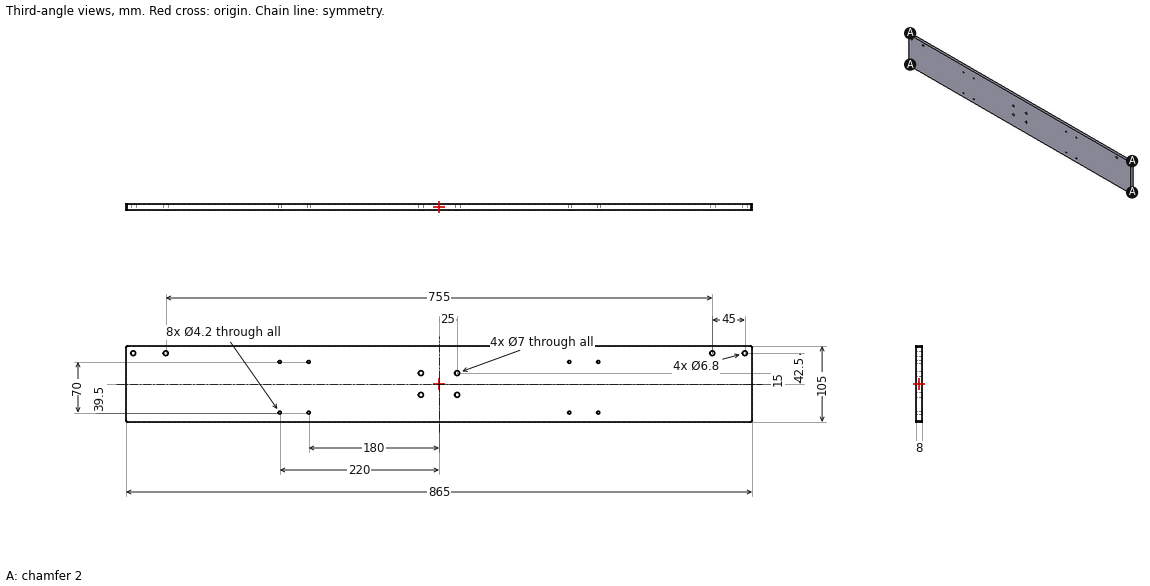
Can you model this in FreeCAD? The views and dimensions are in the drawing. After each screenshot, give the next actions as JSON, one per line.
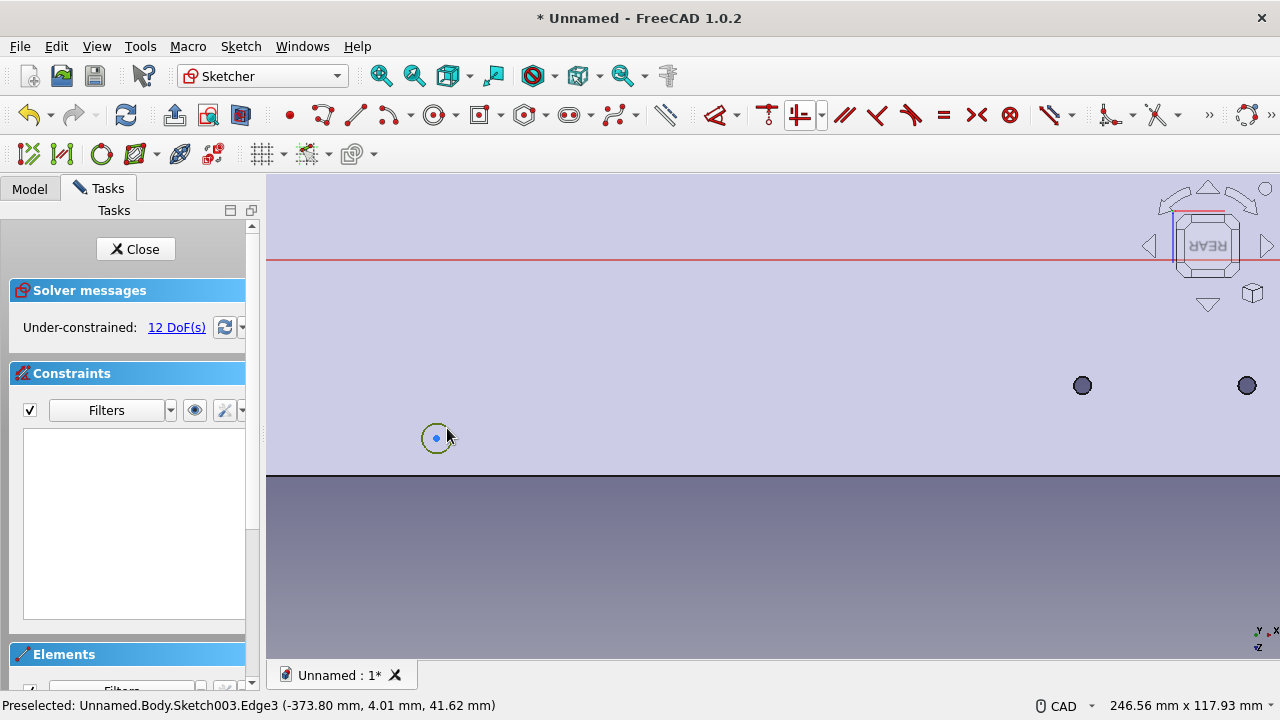
{"action": "scroll", "coordinate": [450, 429], "scroll_direction": "down", "scroll_amount": 9}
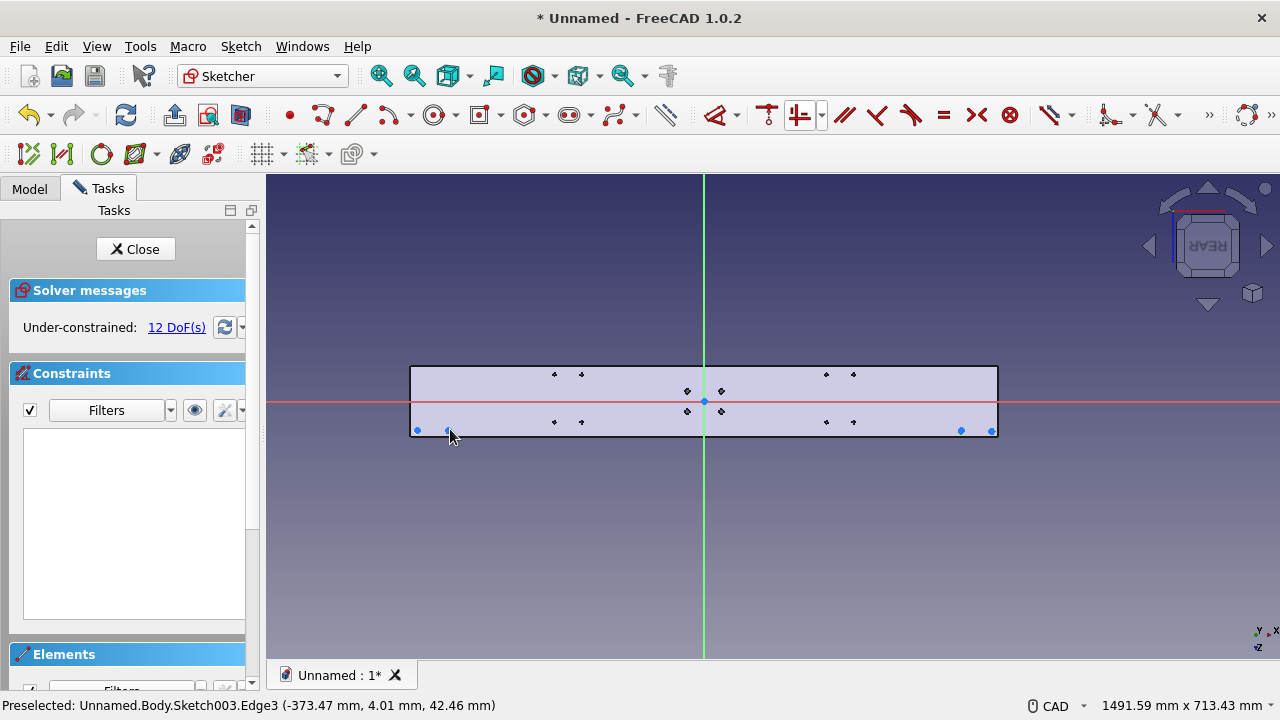
{"action": "scroll", "coordinate": [419, 429], "scroll_direction": "up", "scroll_amount": 9}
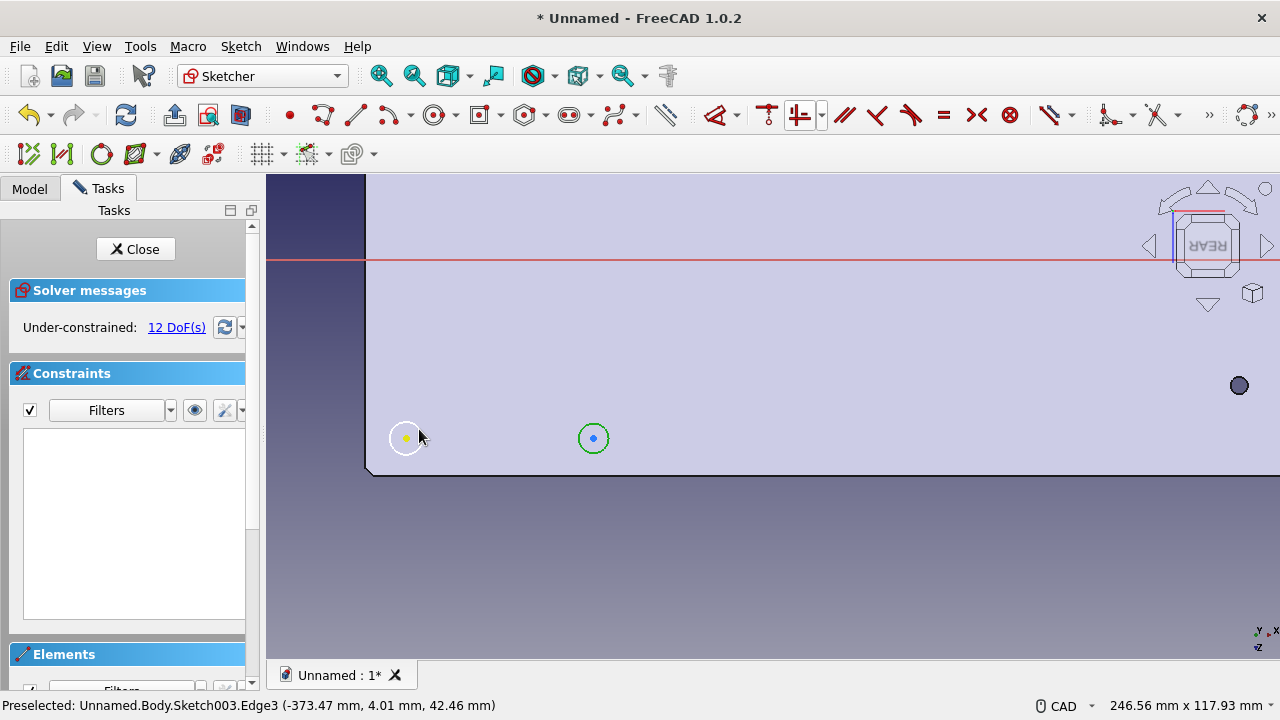
{"action": "left_click", "coordinate": [418, 427]}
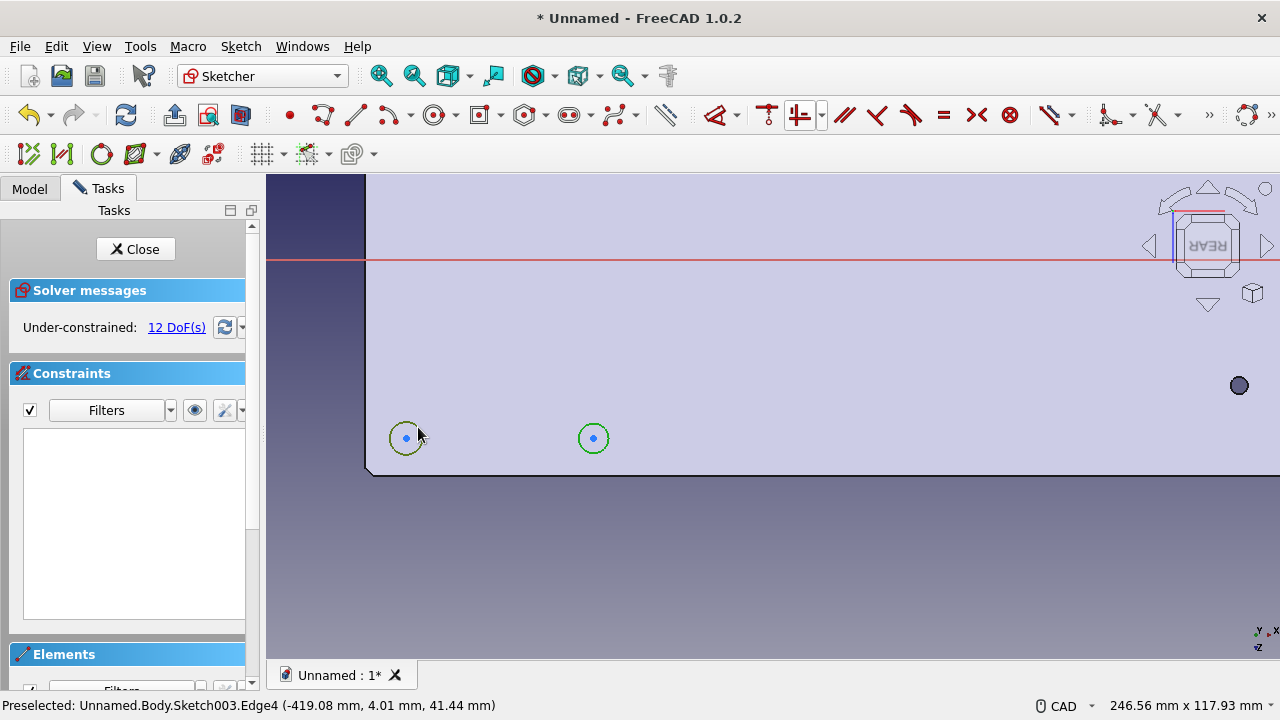
{"action": "key", "text": "e"}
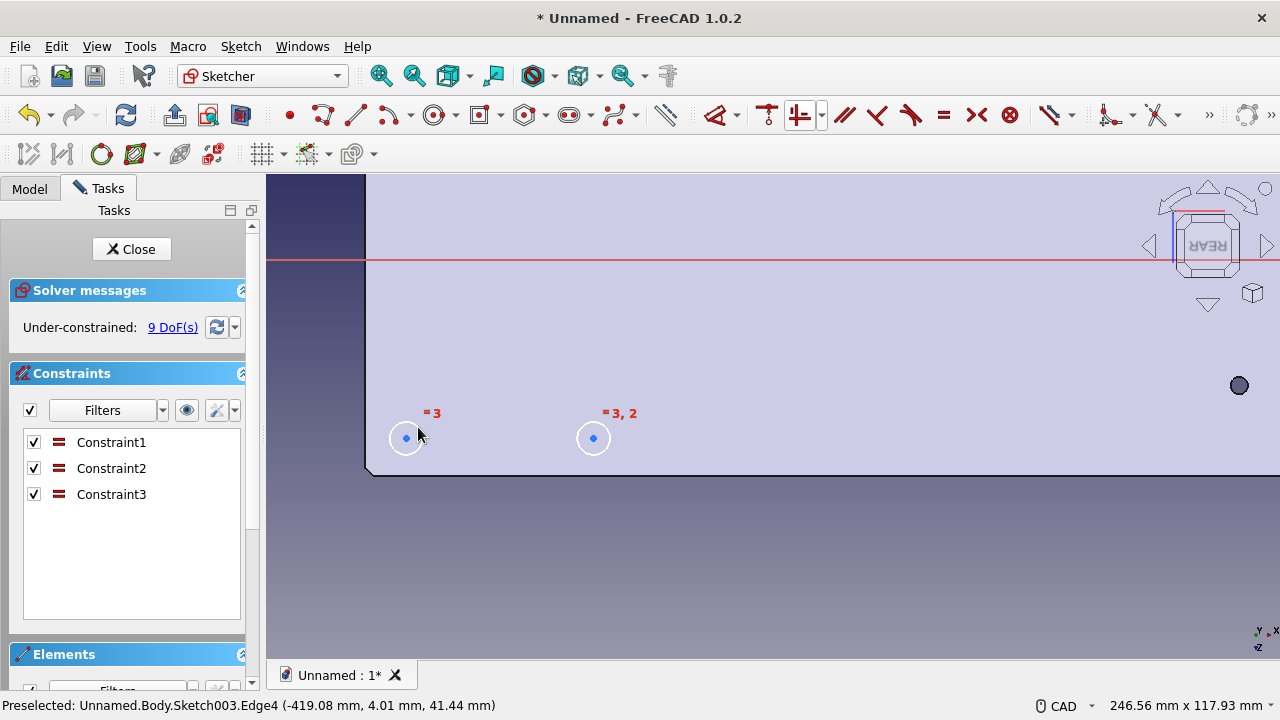
{"action": "scroll", "coordinate": [419, 429], "scroll_direction": "down", "scroll_amount": 9}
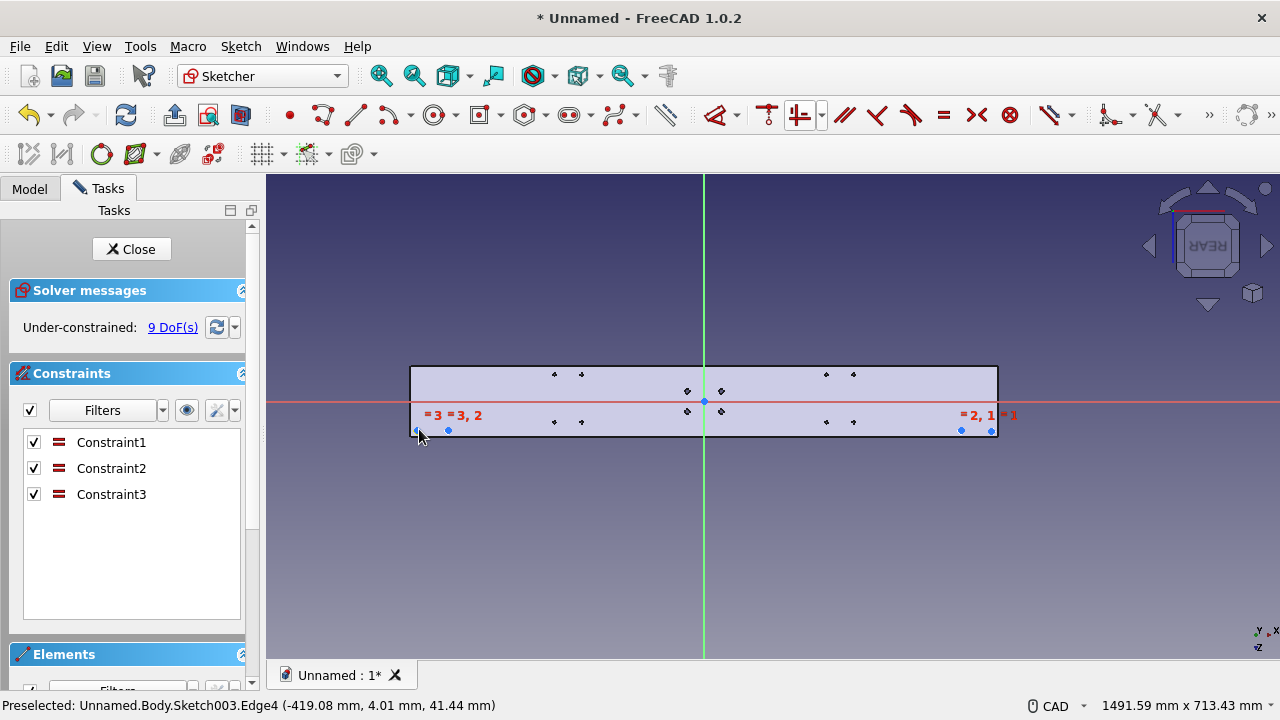
{"action": "left_click", "coordinate": [961, 431]}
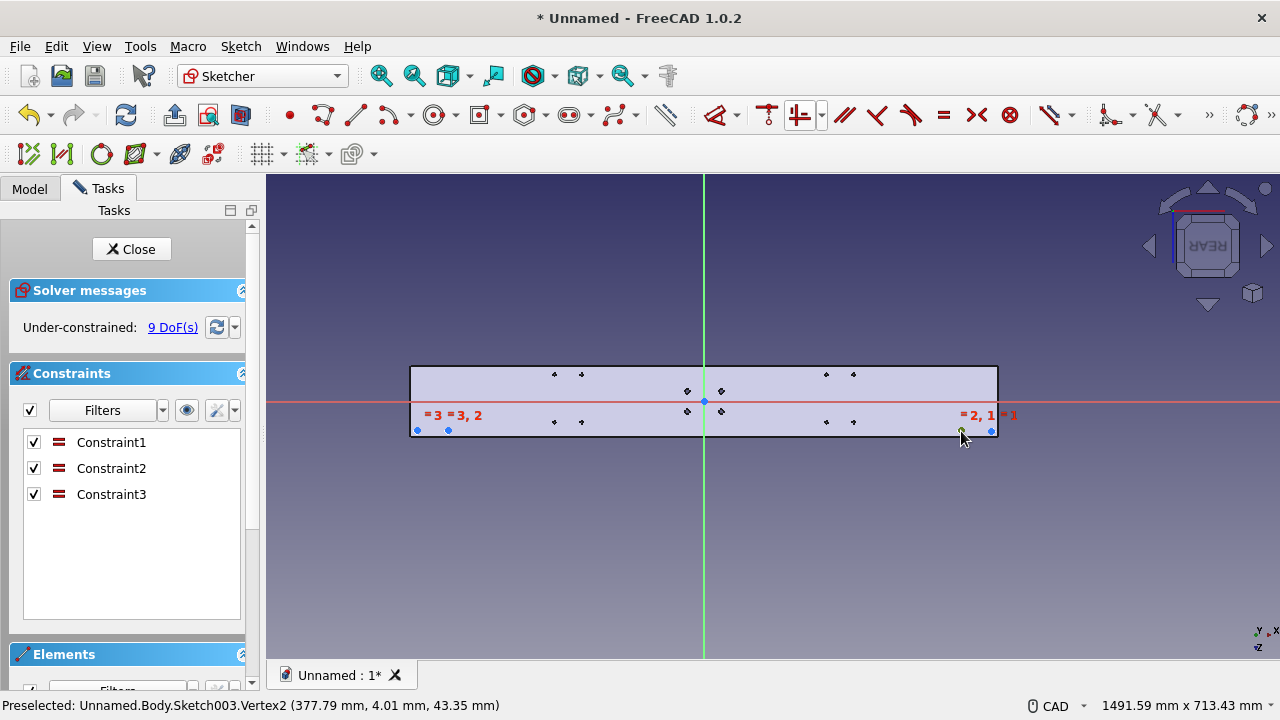
{"action": "left_click", "coordinate": [448, 431]}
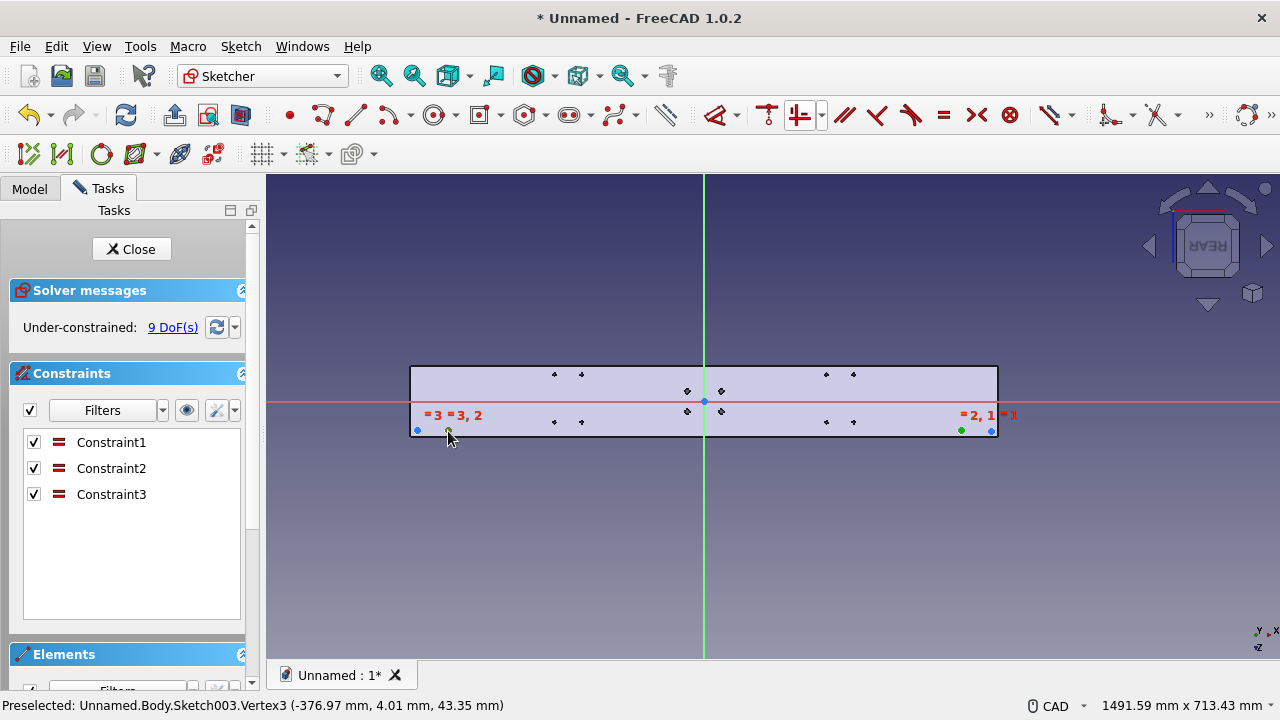
{"action": "left_click", "coordinate": [704, 600]}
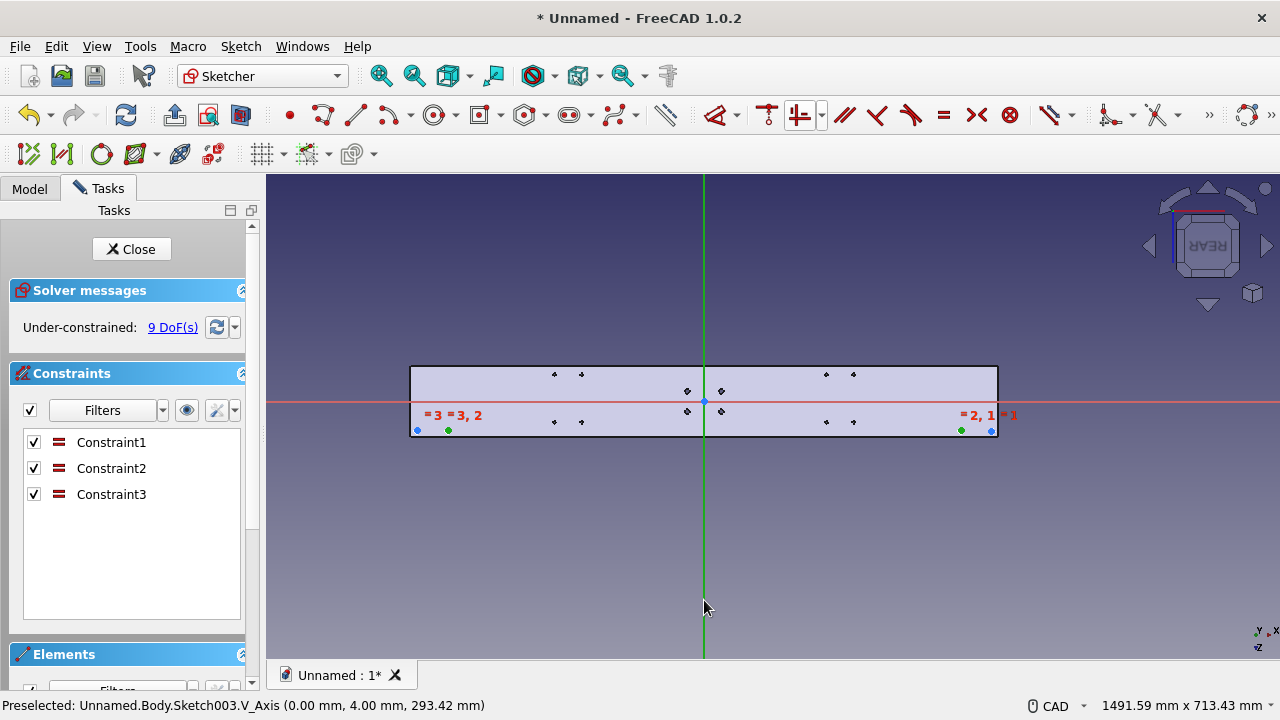
{"action": "left_click", "coordinate": [977, 116]}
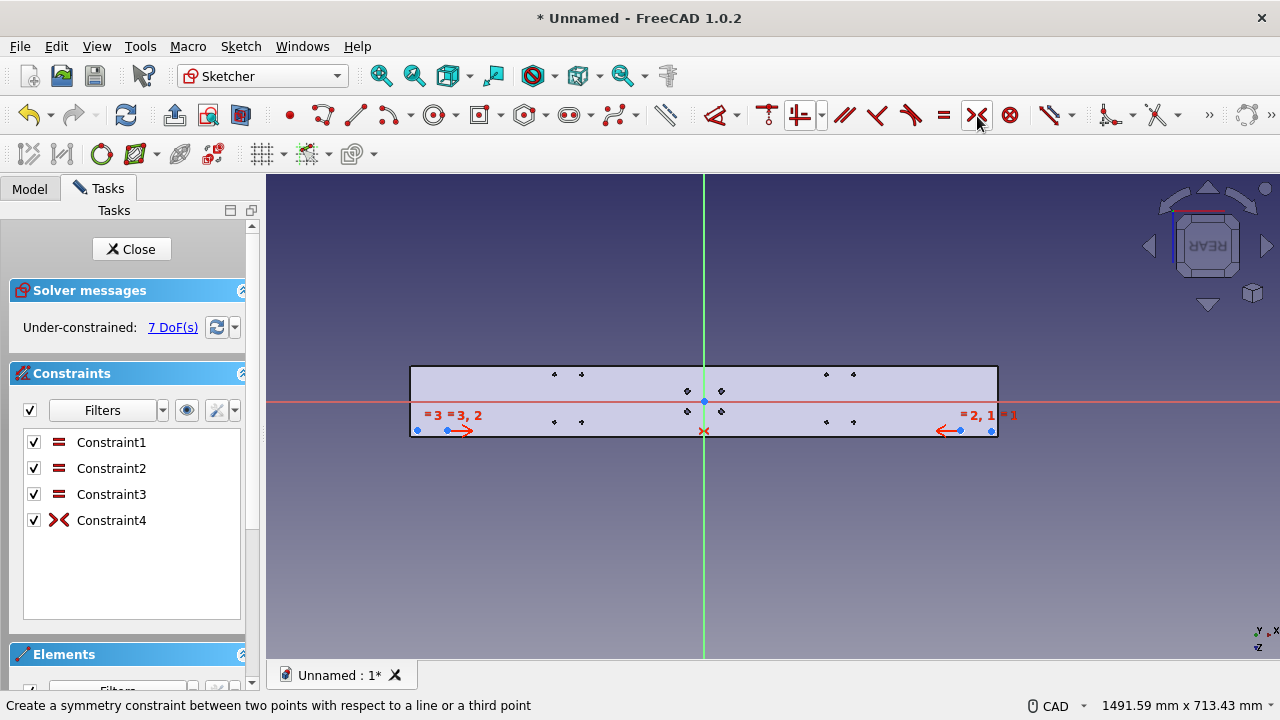
{"action": "left_click", "coordinate": [992, 431]}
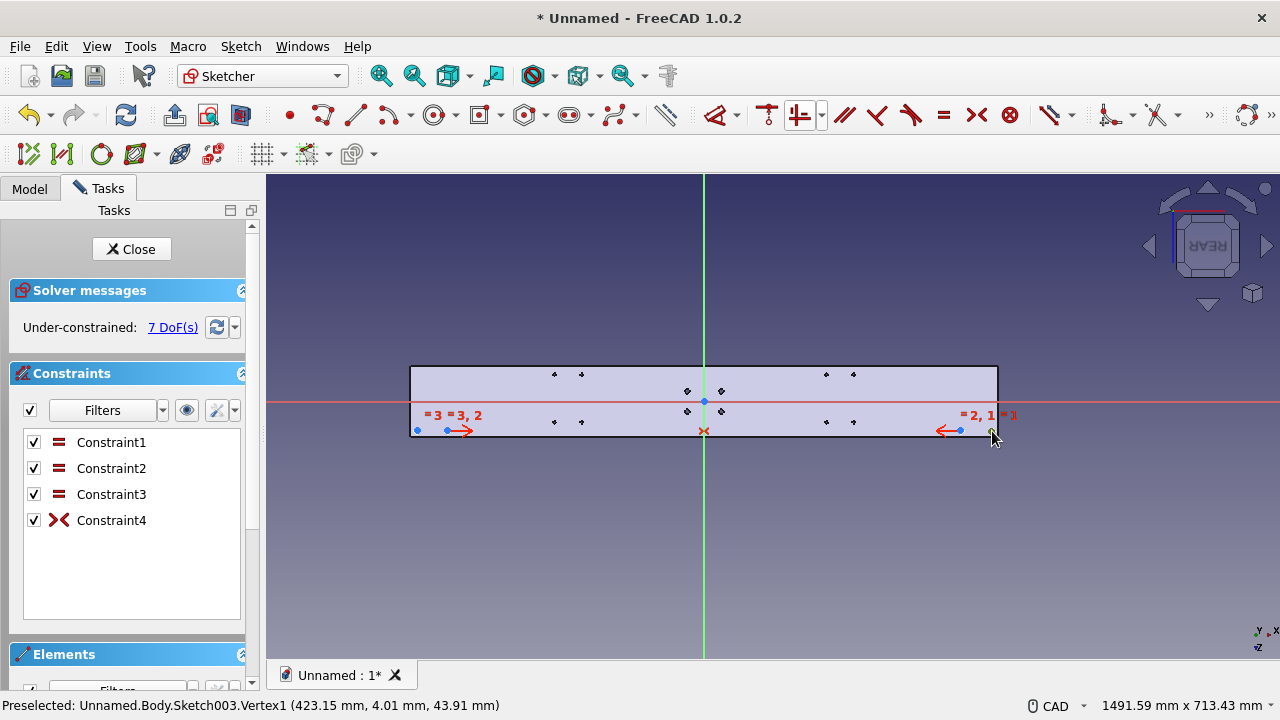
{"action": "left_click", "coordinate": [417, 431]}